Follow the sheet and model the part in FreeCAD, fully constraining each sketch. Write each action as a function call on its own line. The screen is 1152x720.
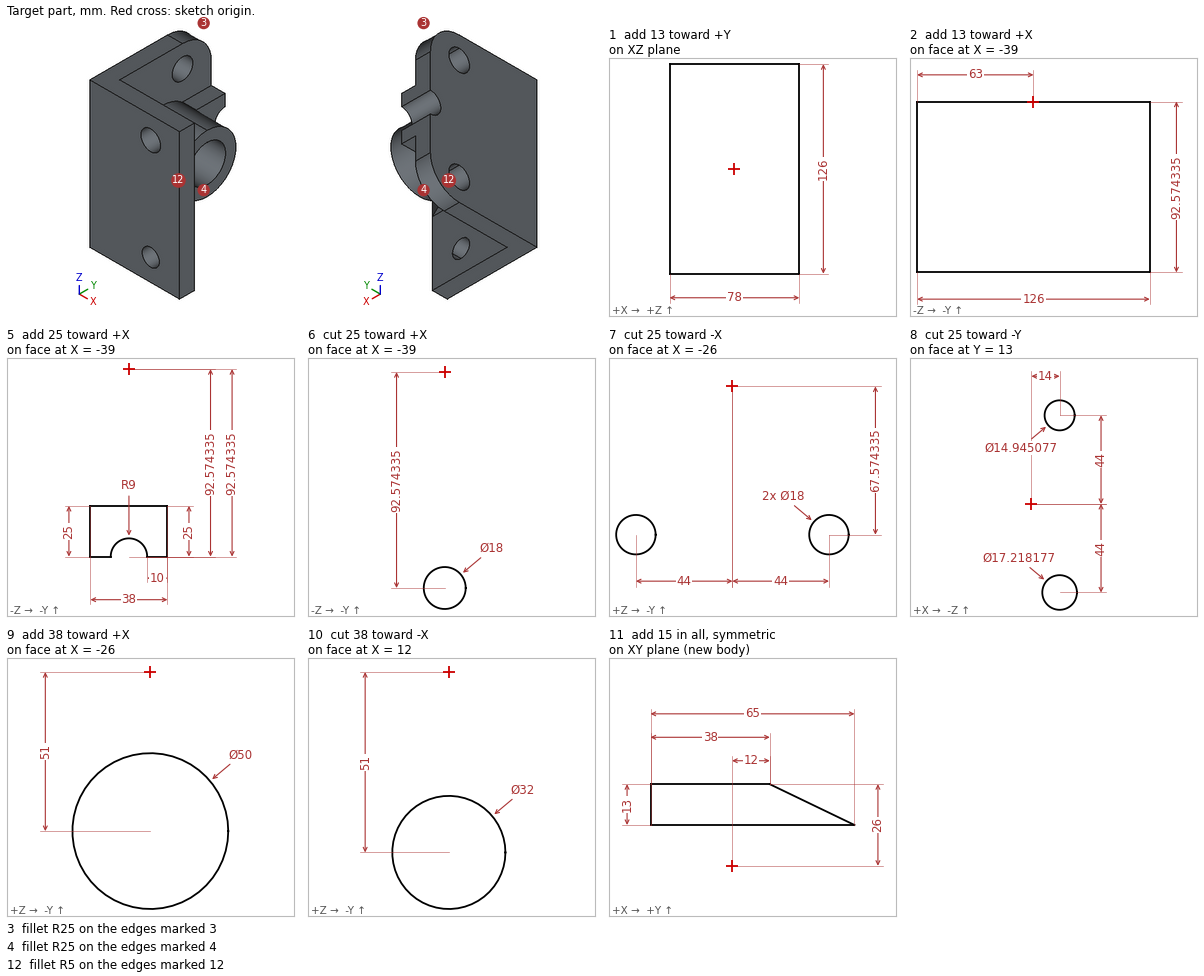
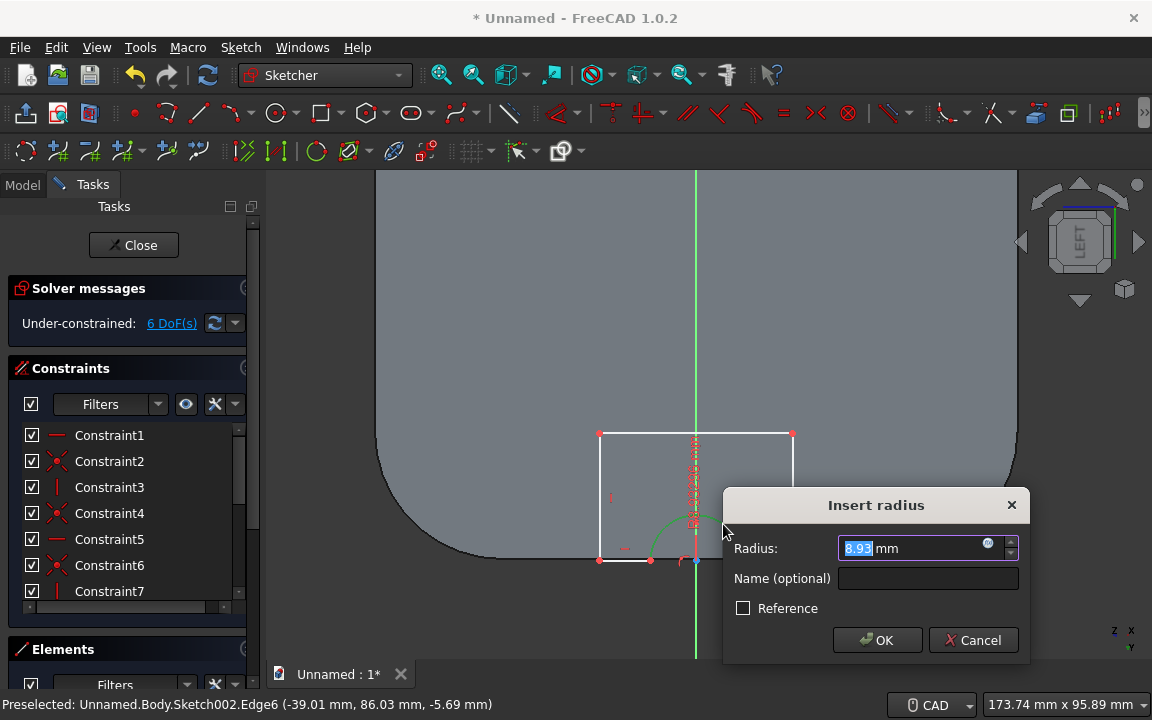
text(9)
key(Return)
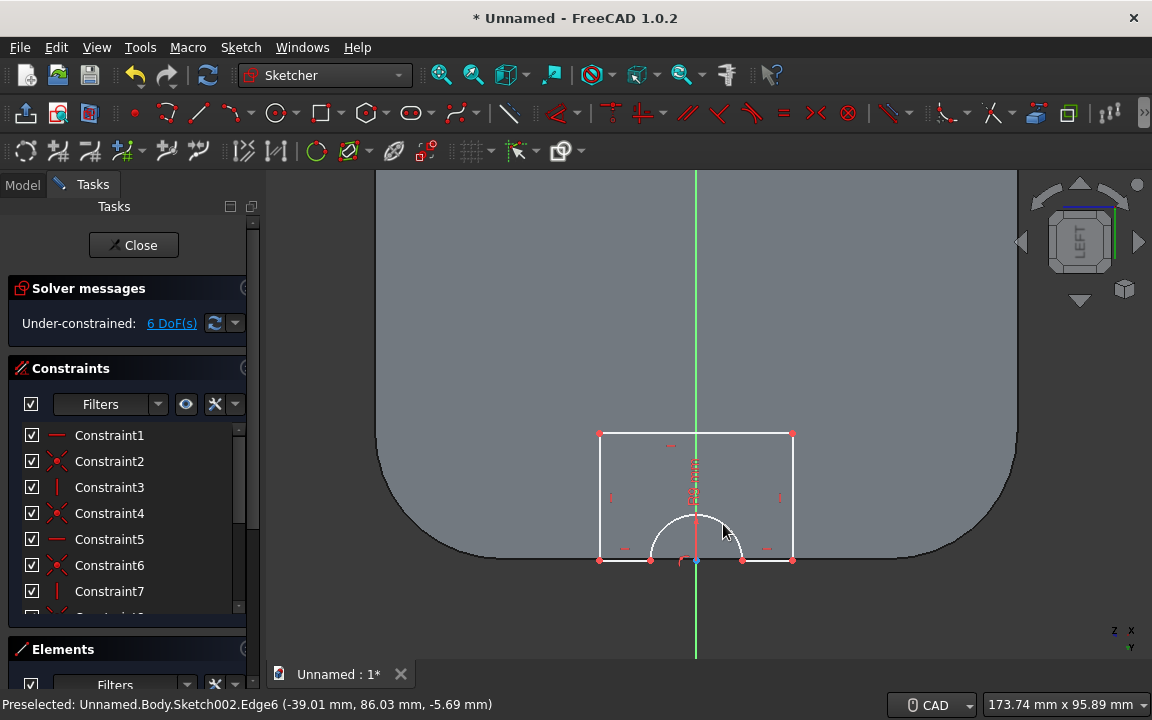
click(757, 561)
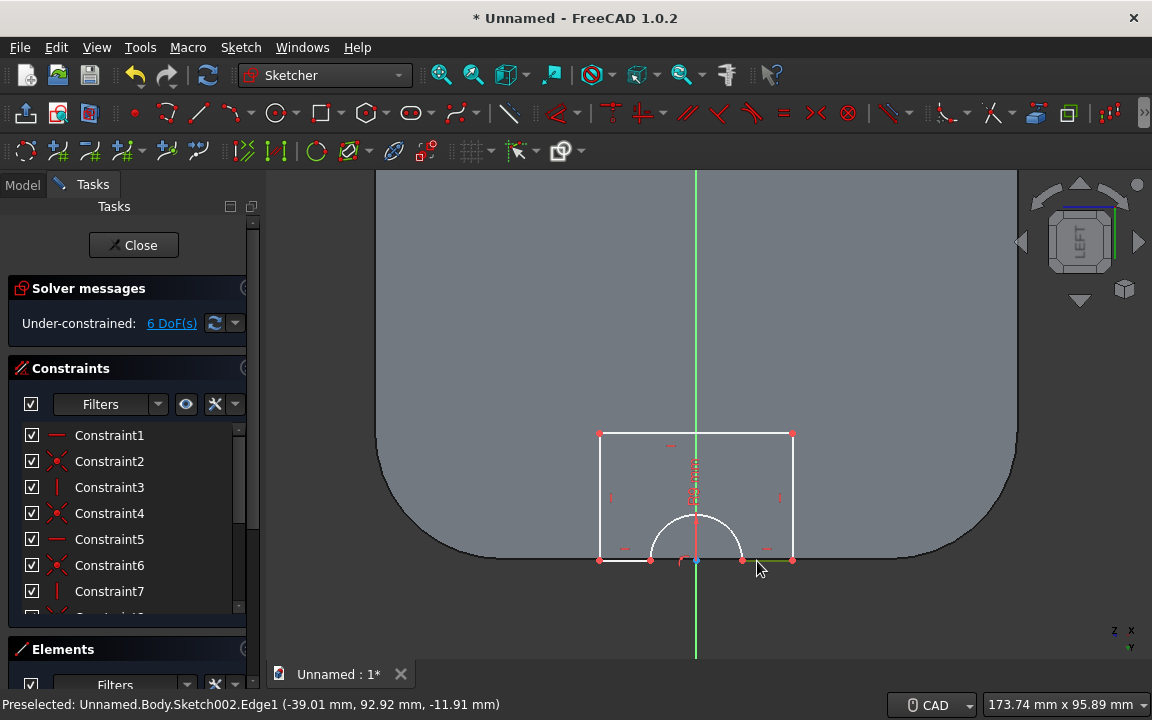
key(l)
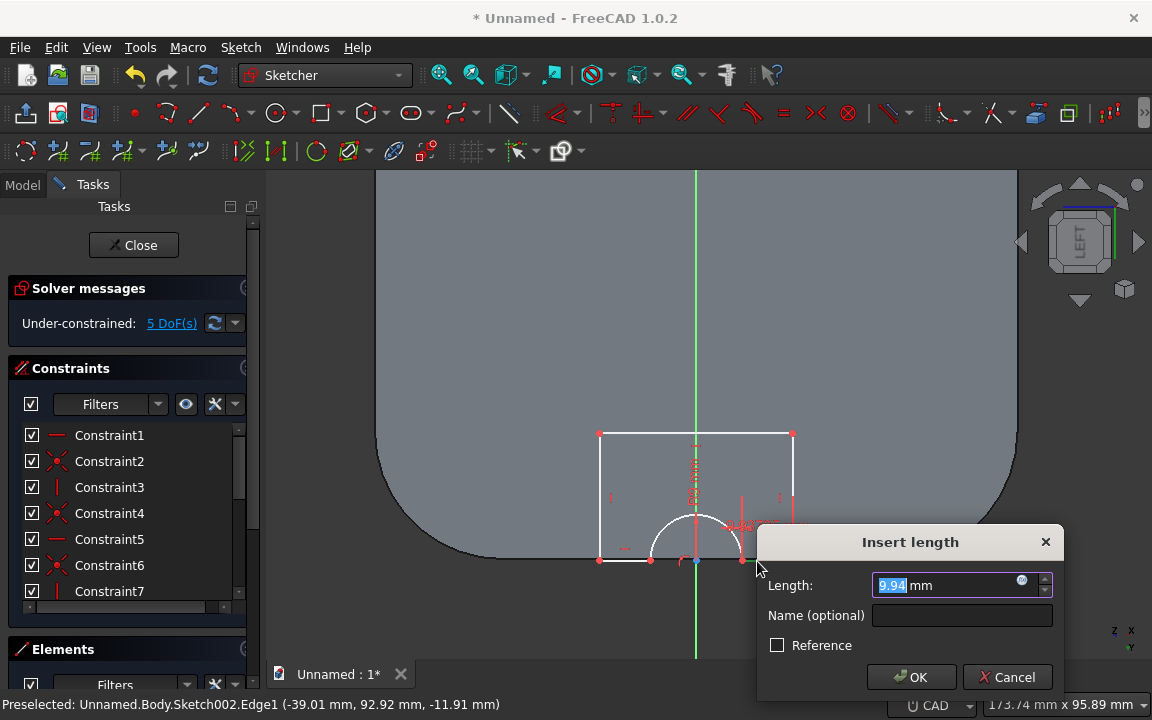
text(10)
key(Return)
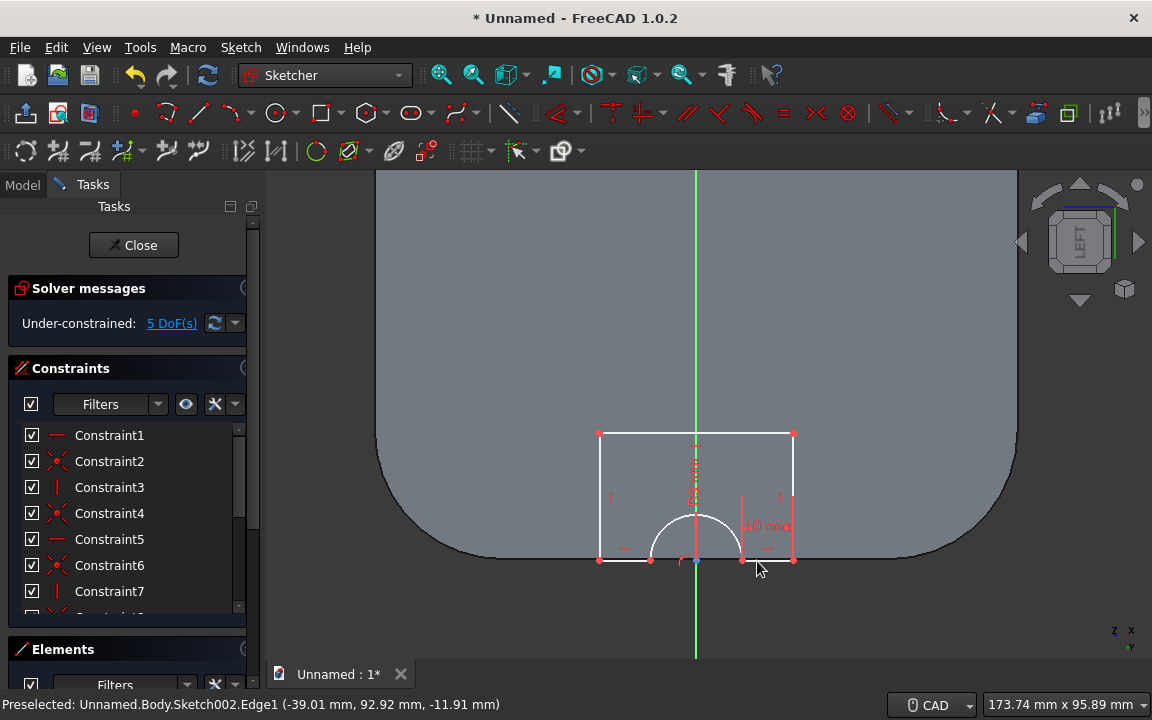
click(793, 523)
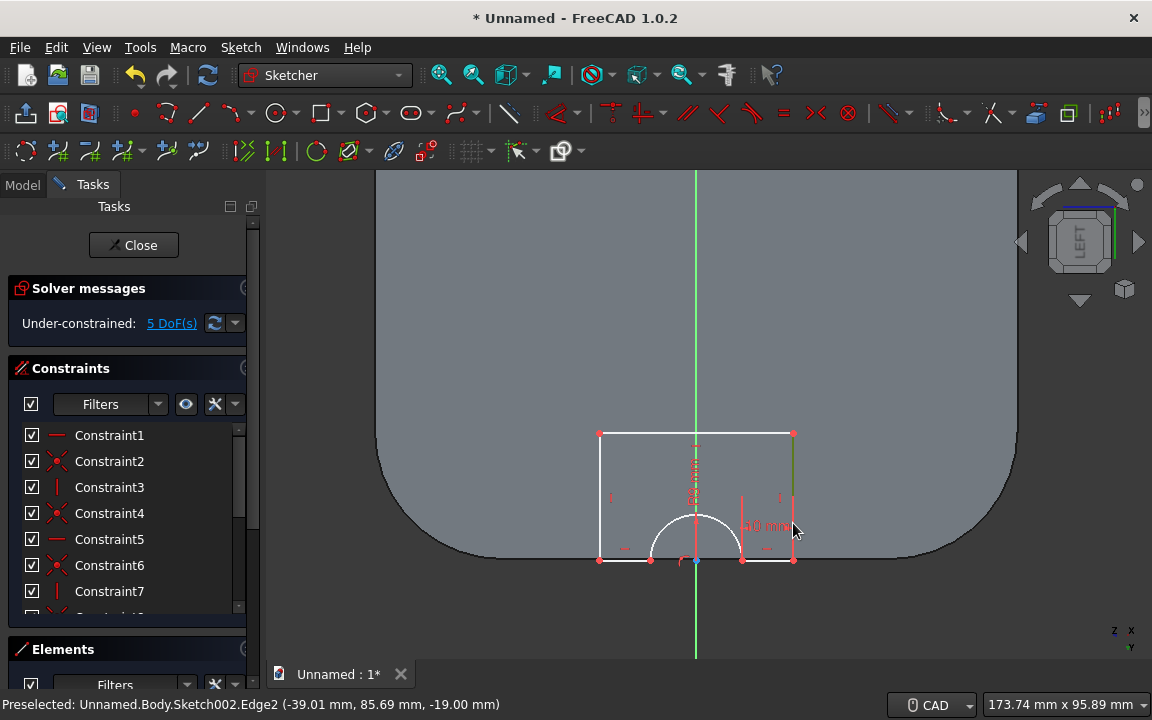
key(i)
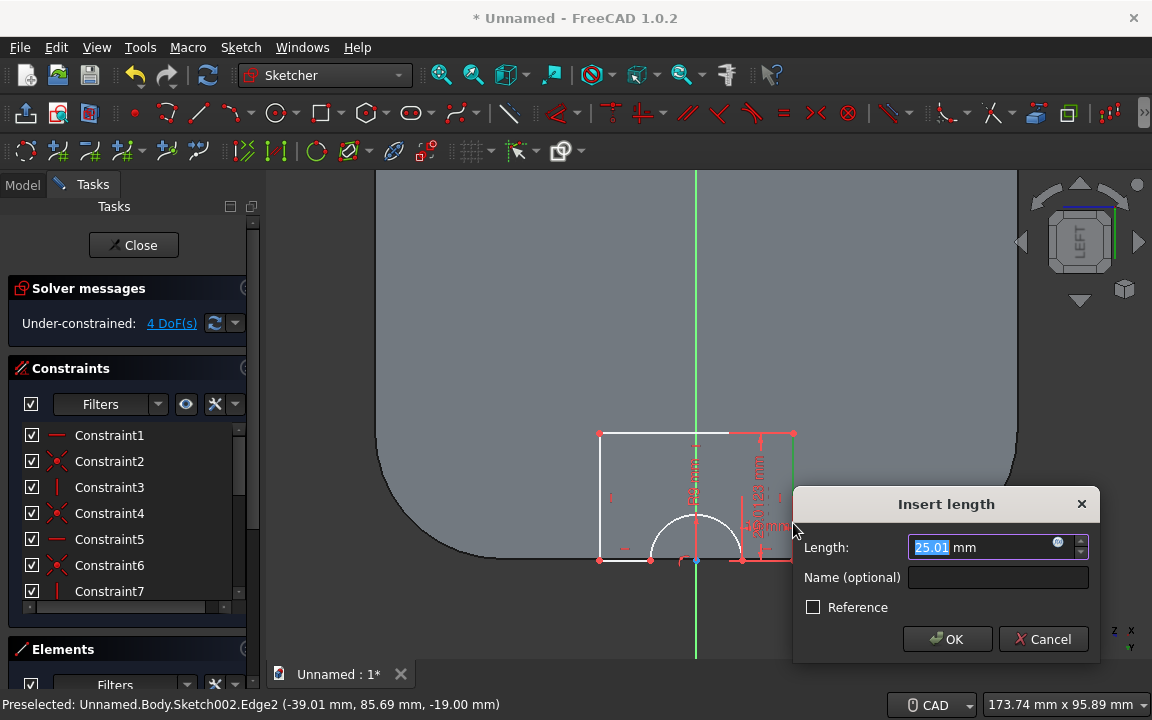
text(25)
key(Return)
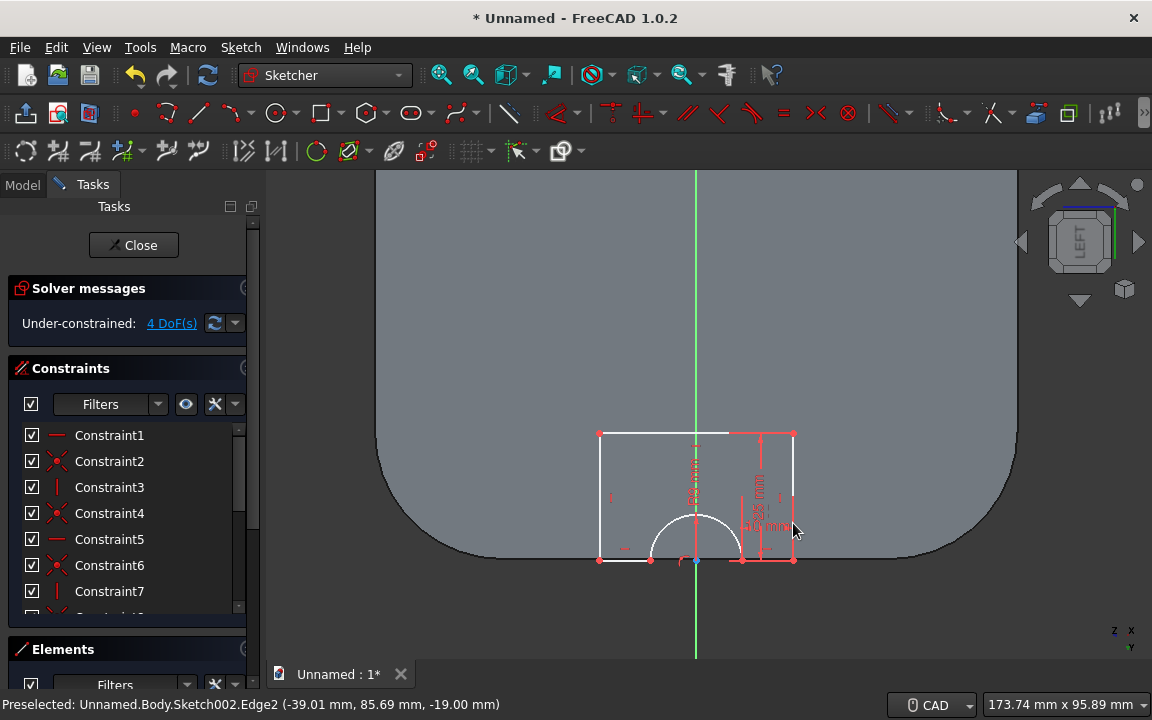
click(735, 433)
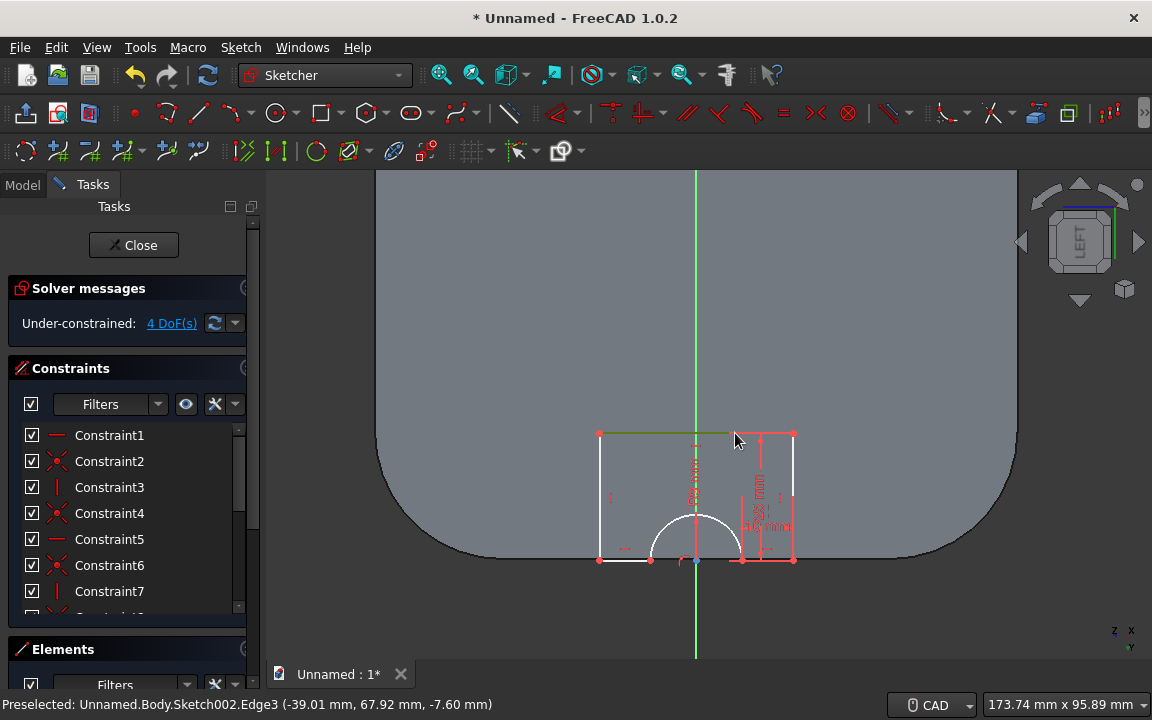
key(l)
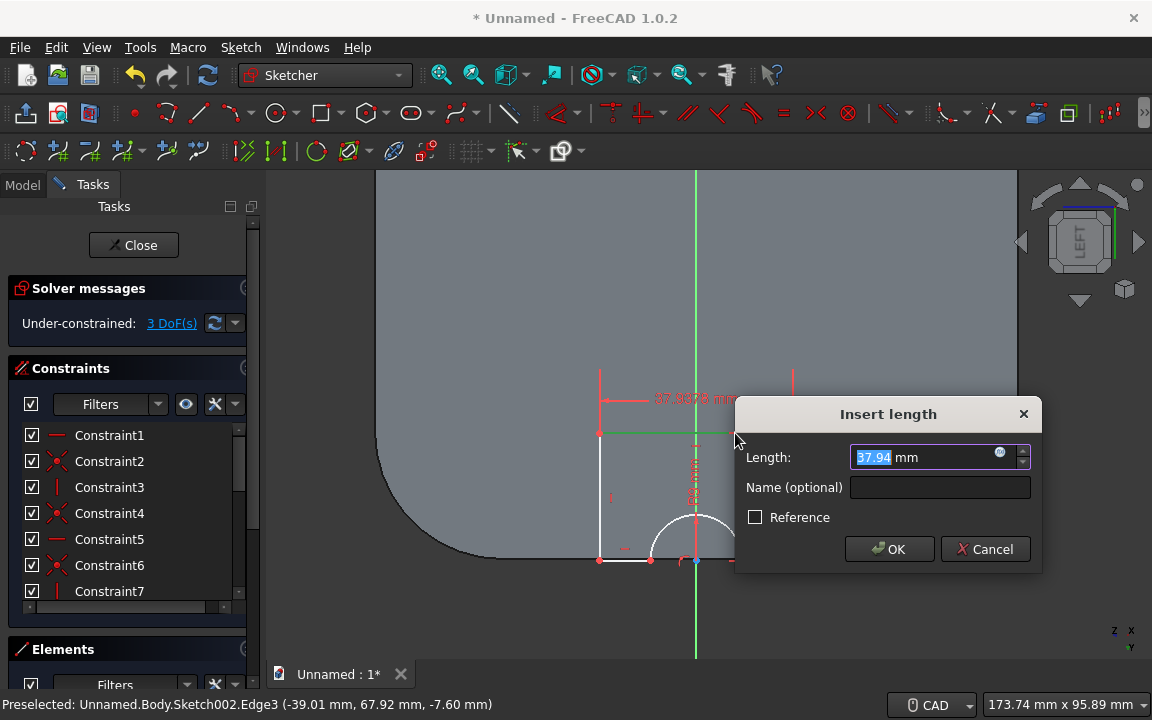
text(38)
key(Return)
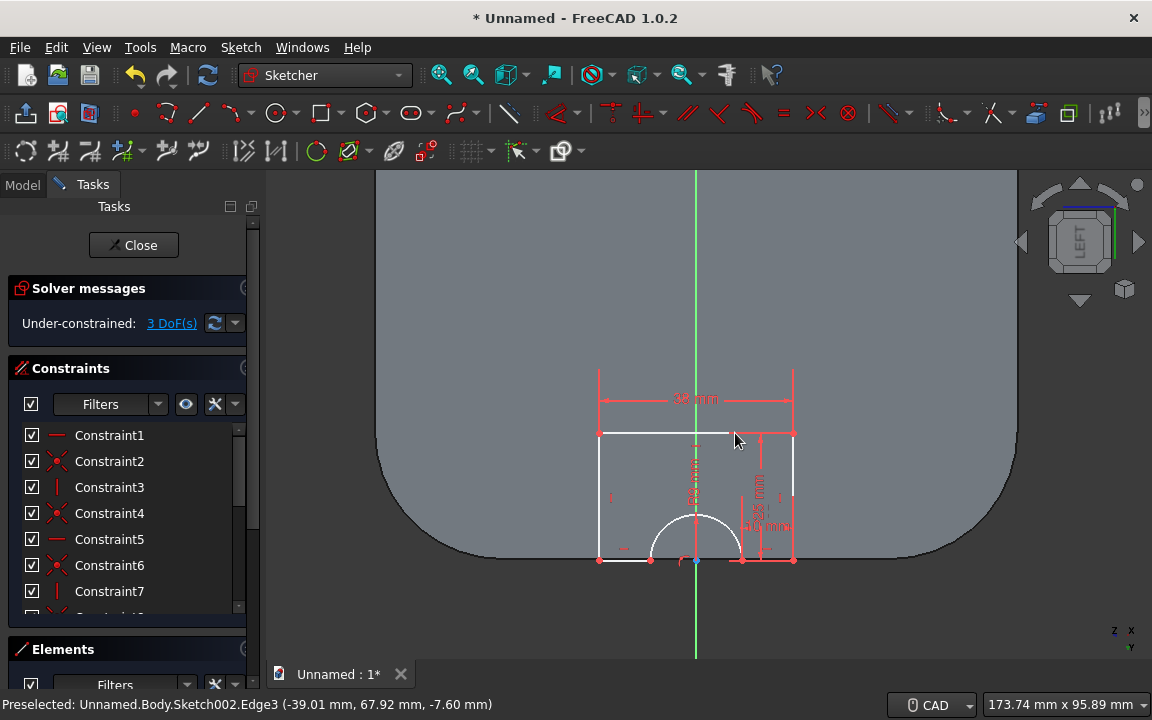
click(599, 472)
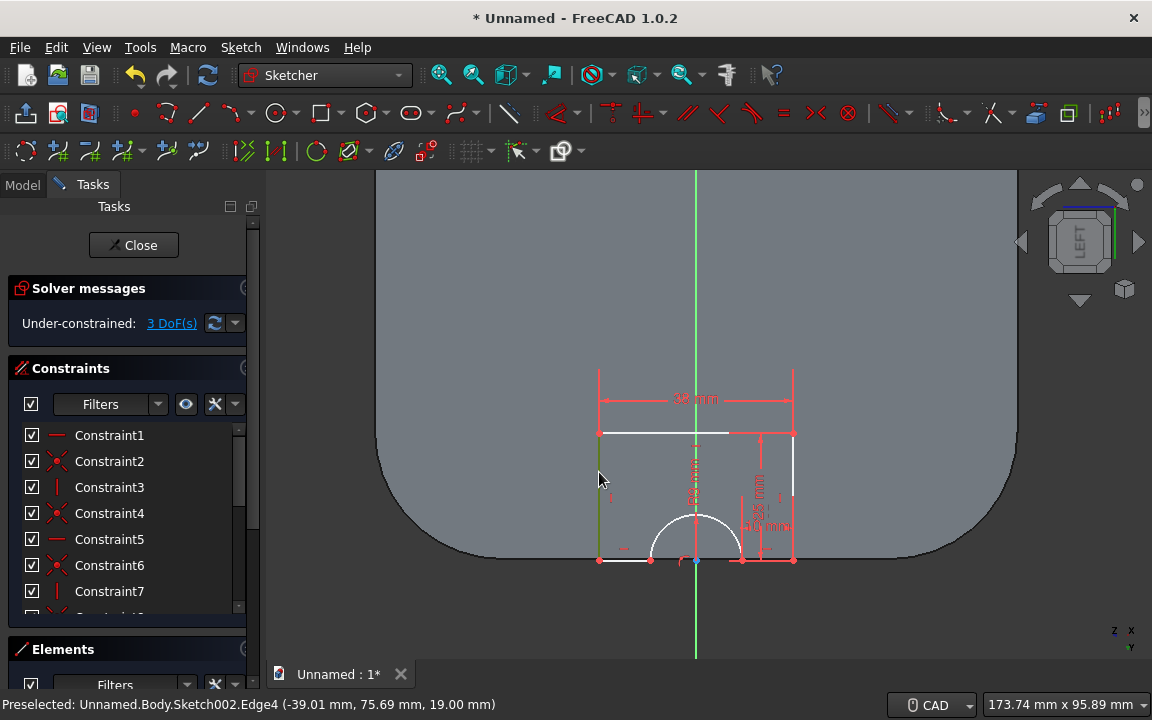
key(i)